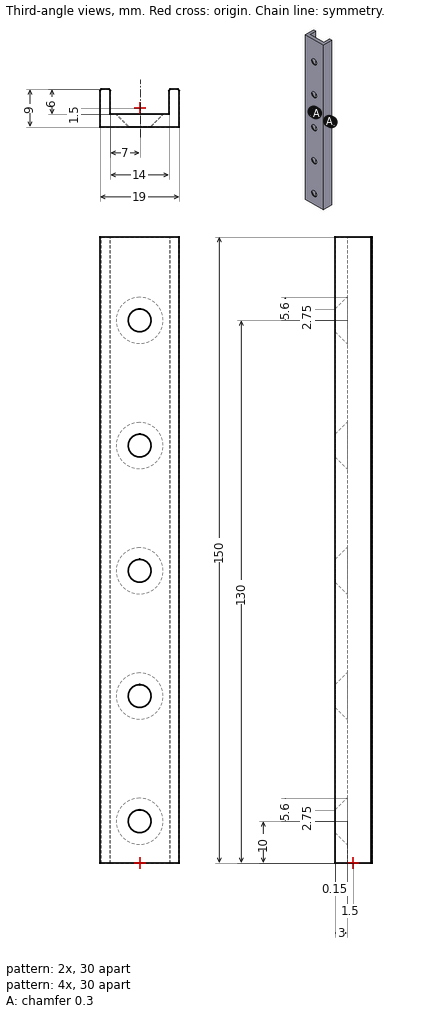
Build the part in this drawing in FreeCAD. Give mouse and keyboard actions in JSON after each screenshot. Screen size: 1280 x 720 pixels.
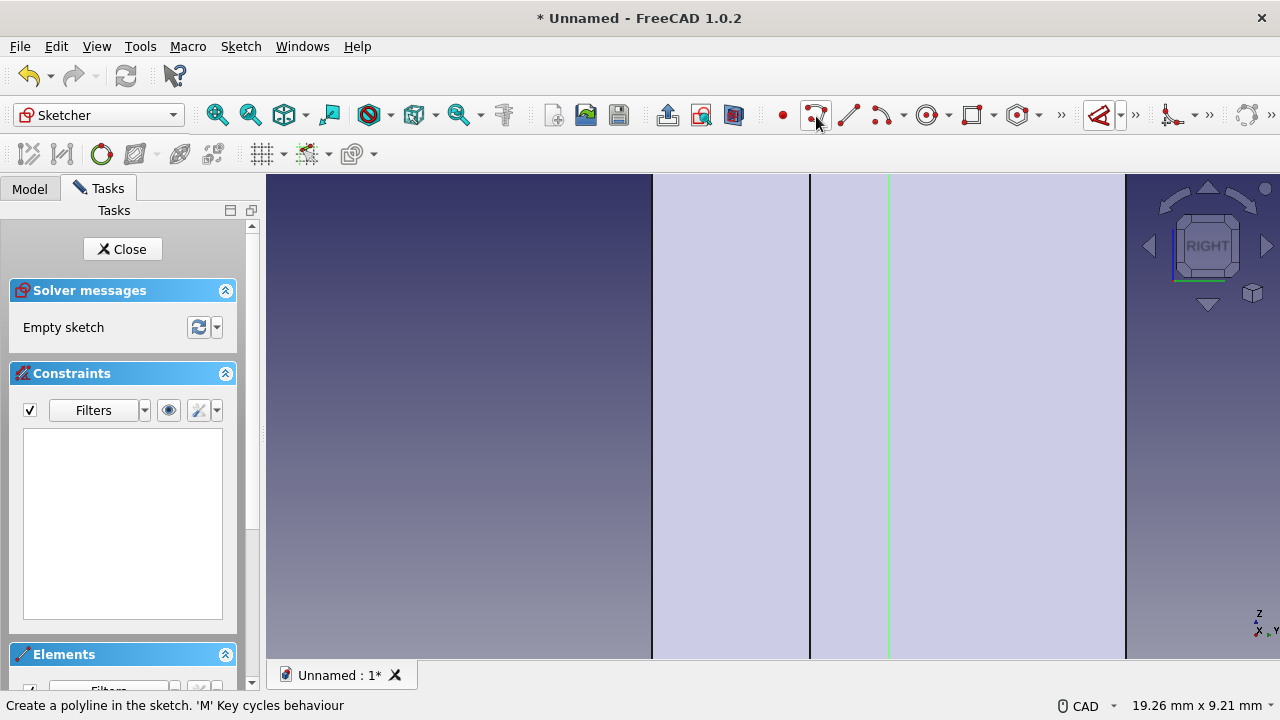
{"action": "left_click", "coordinate": [810, 569]}
{"action": "left_click", "coordinate": [810, 274]}
{"action": "left_click", "coordinate": [660, 424]}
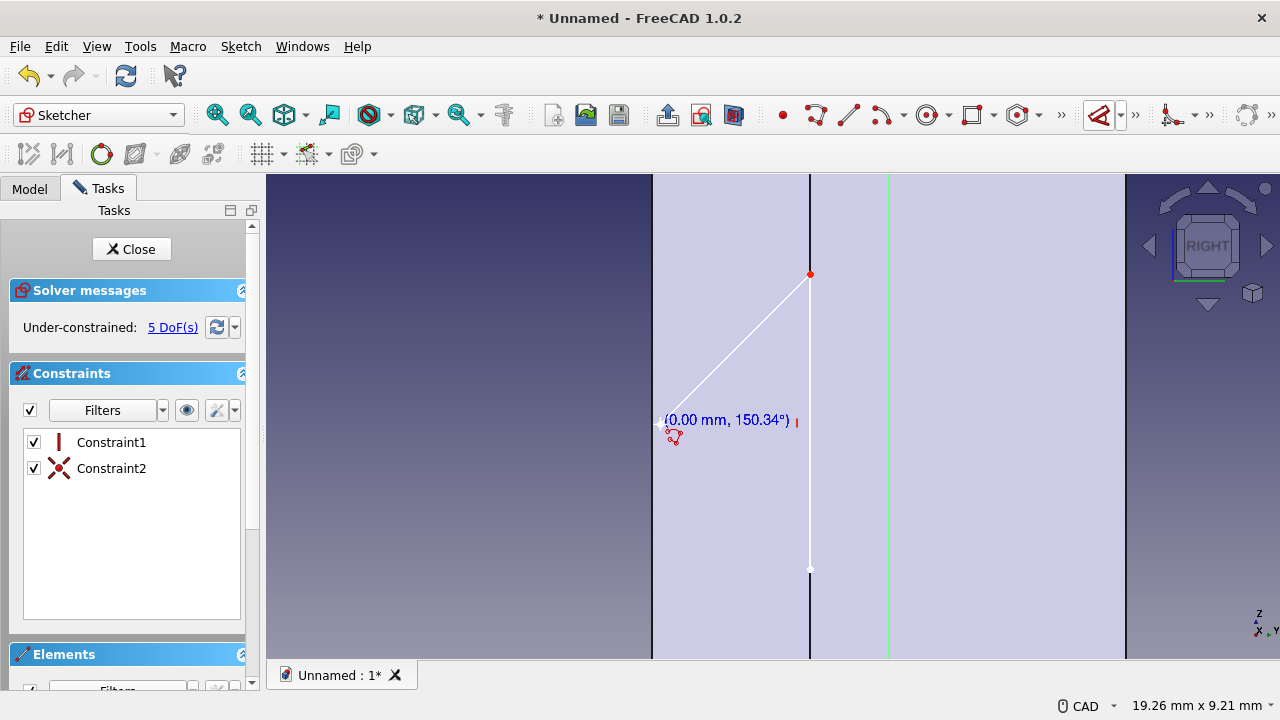
{"action": "scroll", "coordinate": [652, 424], "scroll_direction": "up", "scroll_amount": 4}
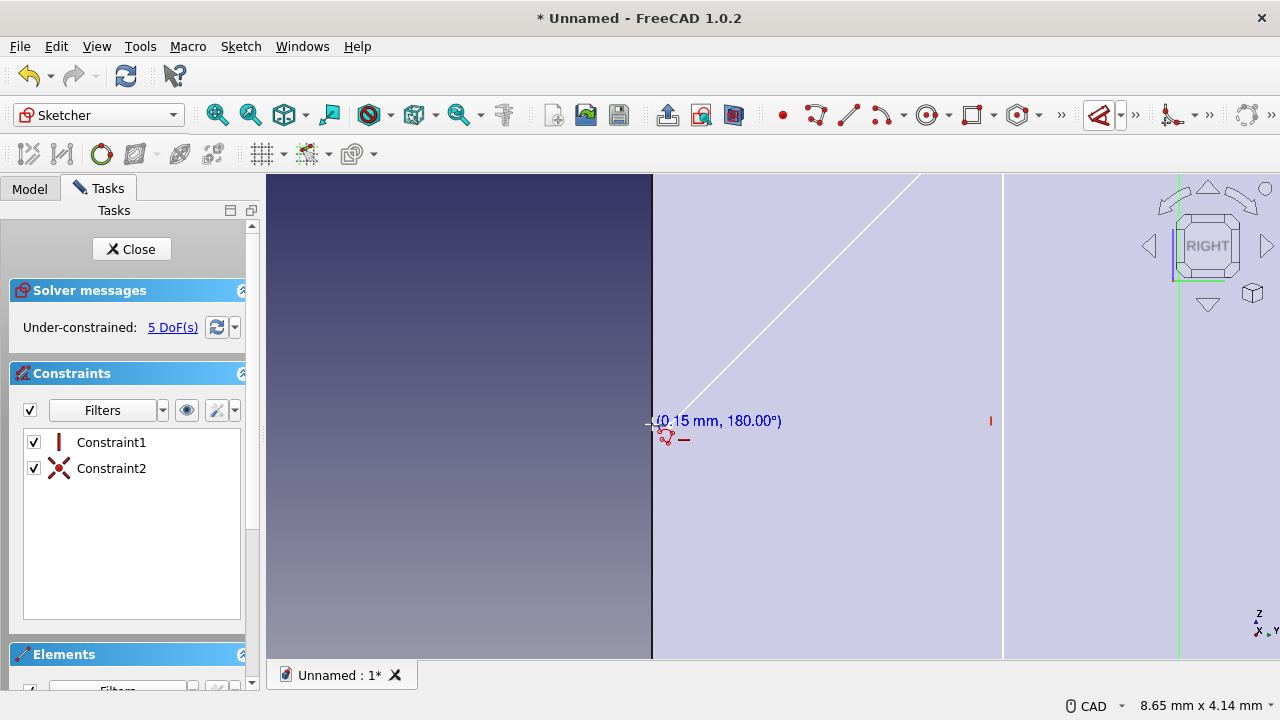
{"action": "left_click", "coordinate": [652, 423]}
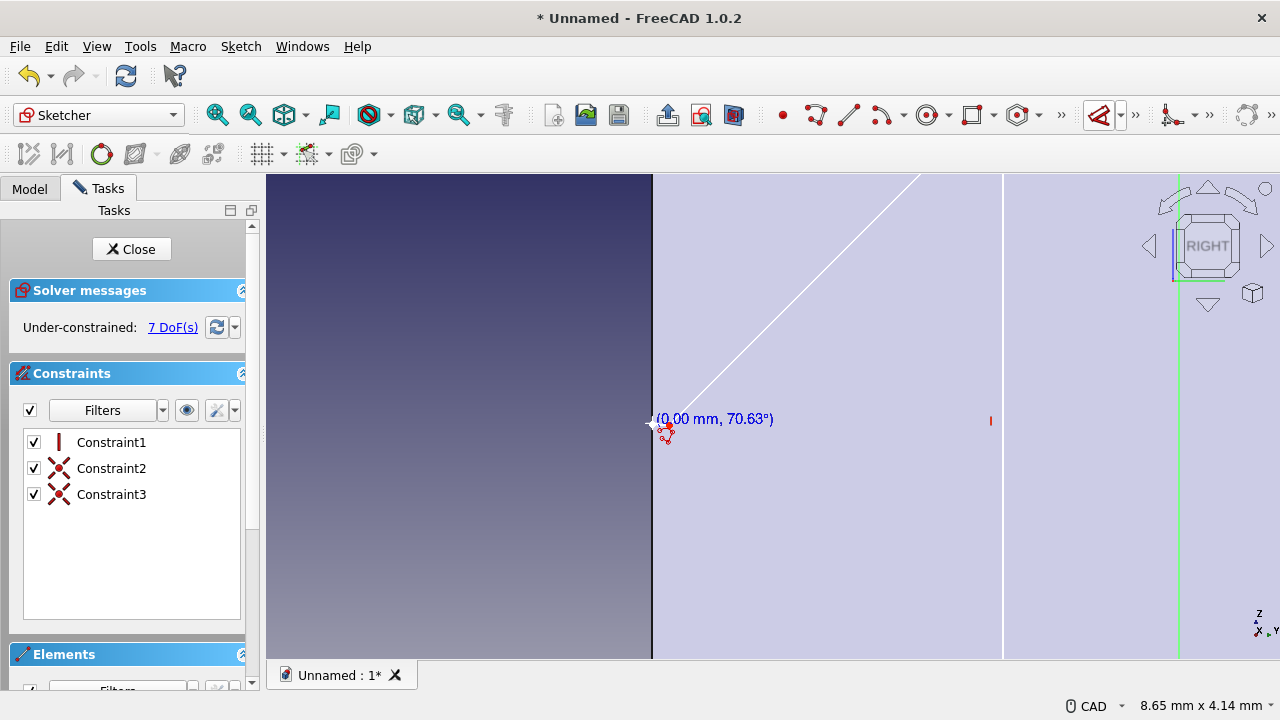
{"action": "scroll", "coordinate": [662, 415], "scroll_direction": "down", "scroll_amount": 4}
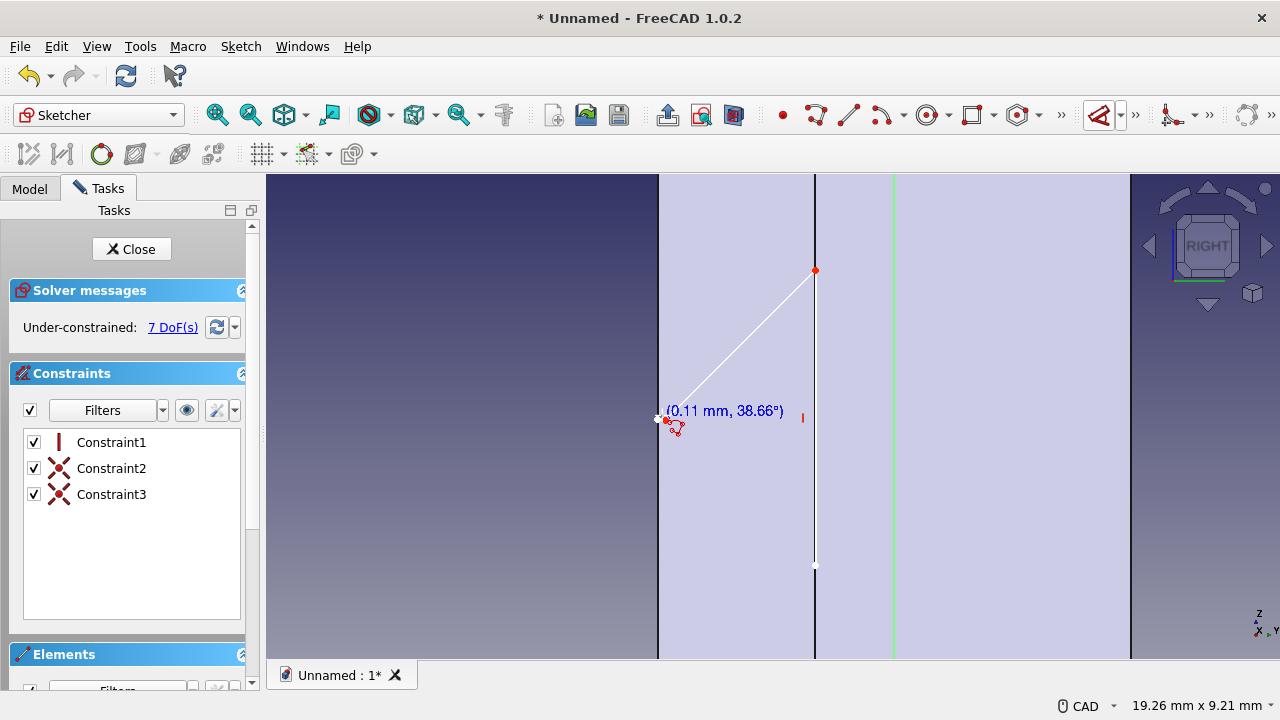
{"action": "left_click", "coordinate": [658, 564]}
{"action": "left_click", "coordinate": [816, 565]}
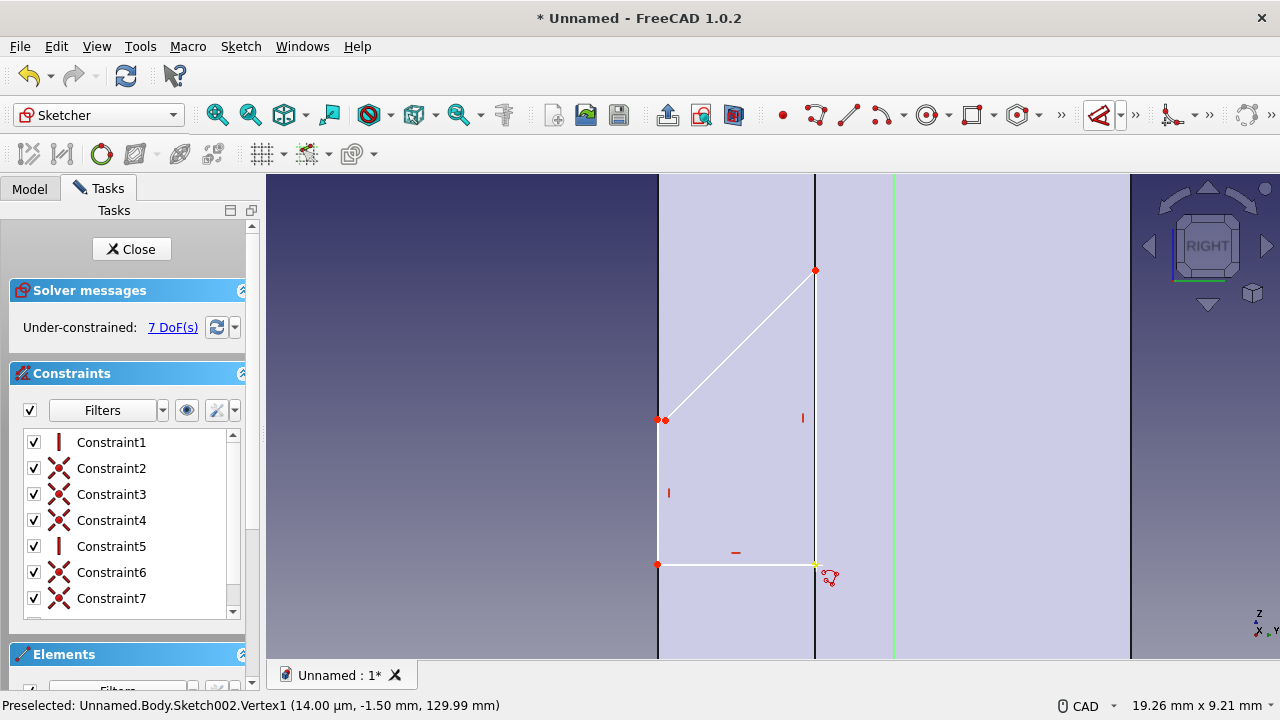
{"action": "left_click", "coordinate": [849, 116]}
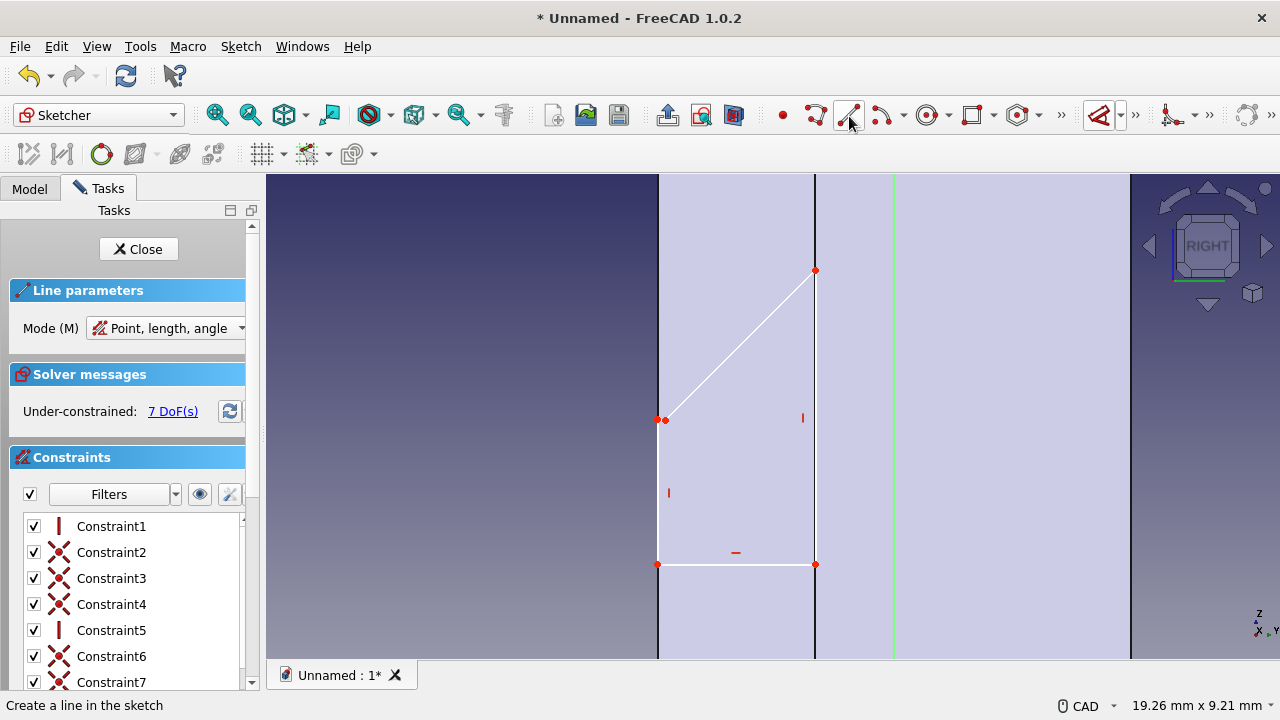
{"action": "left_click", "coordinate": [642, 564]}
{"action": "left_click", "coordinate": [594, 564]}
{"action": "key", "text": "Escape"}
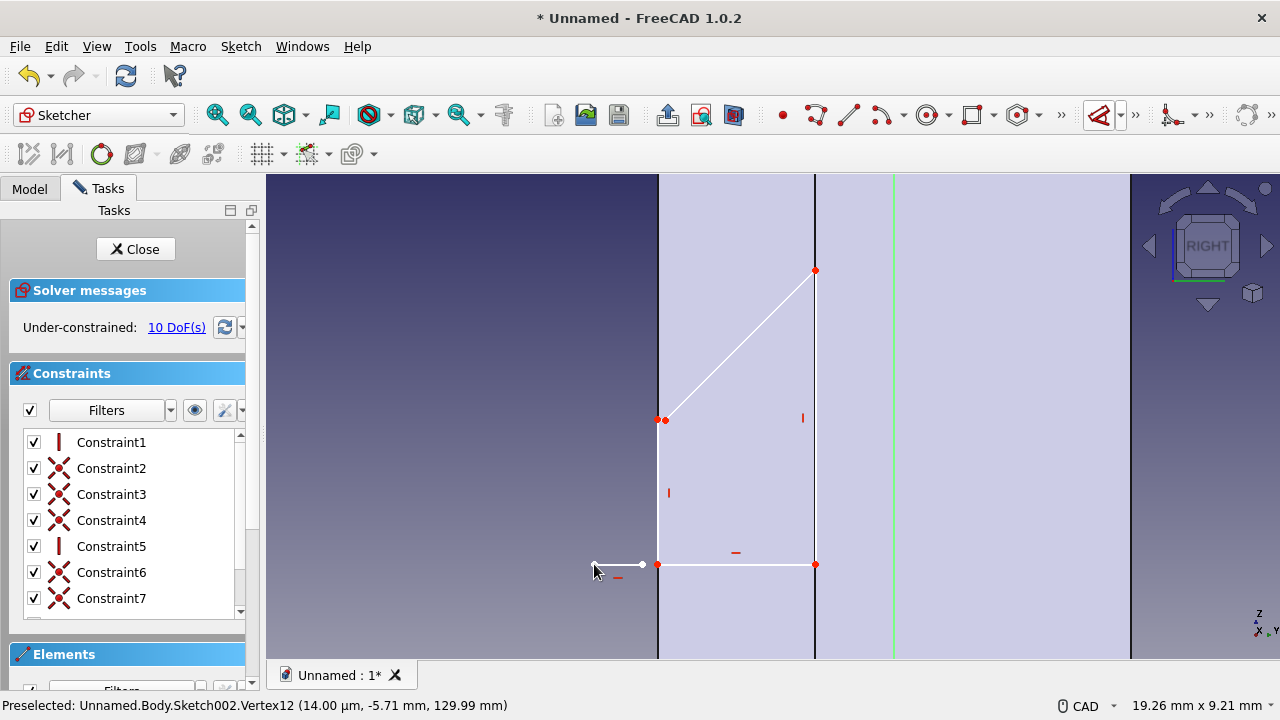
{"action": "left_click", "coordinate": [628, 565]}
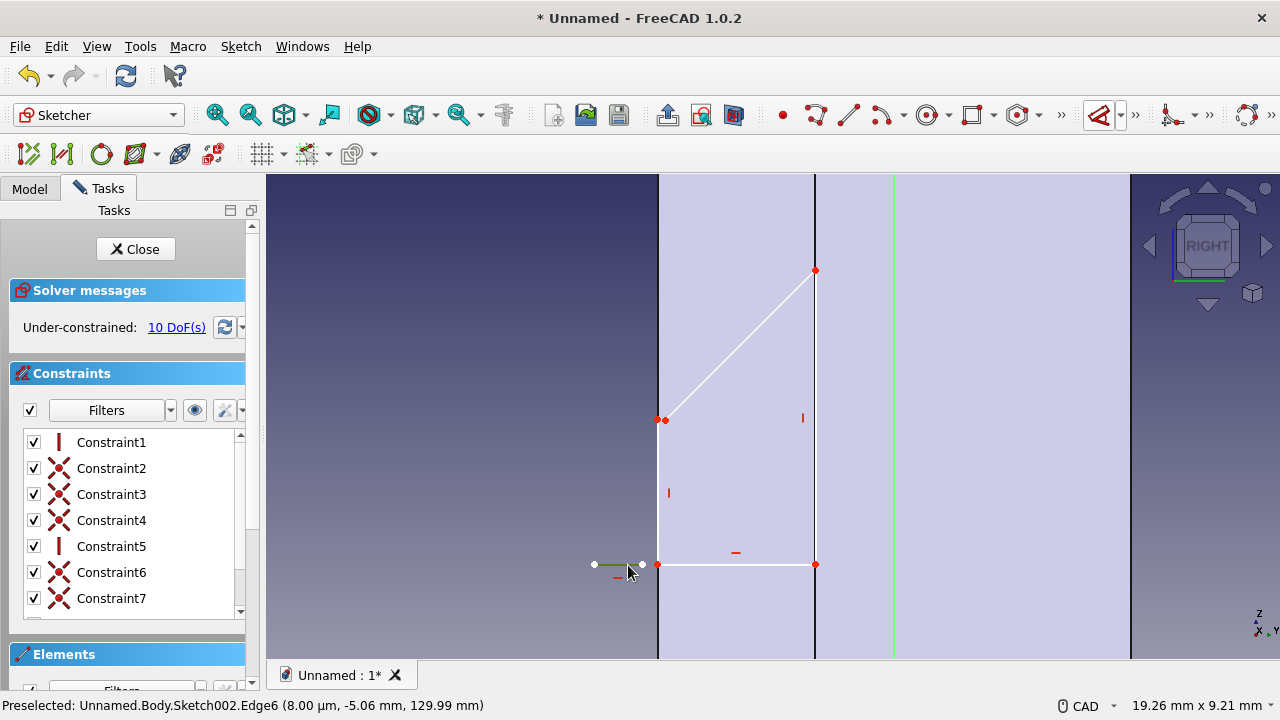
{"action": "key", "text": "g n"}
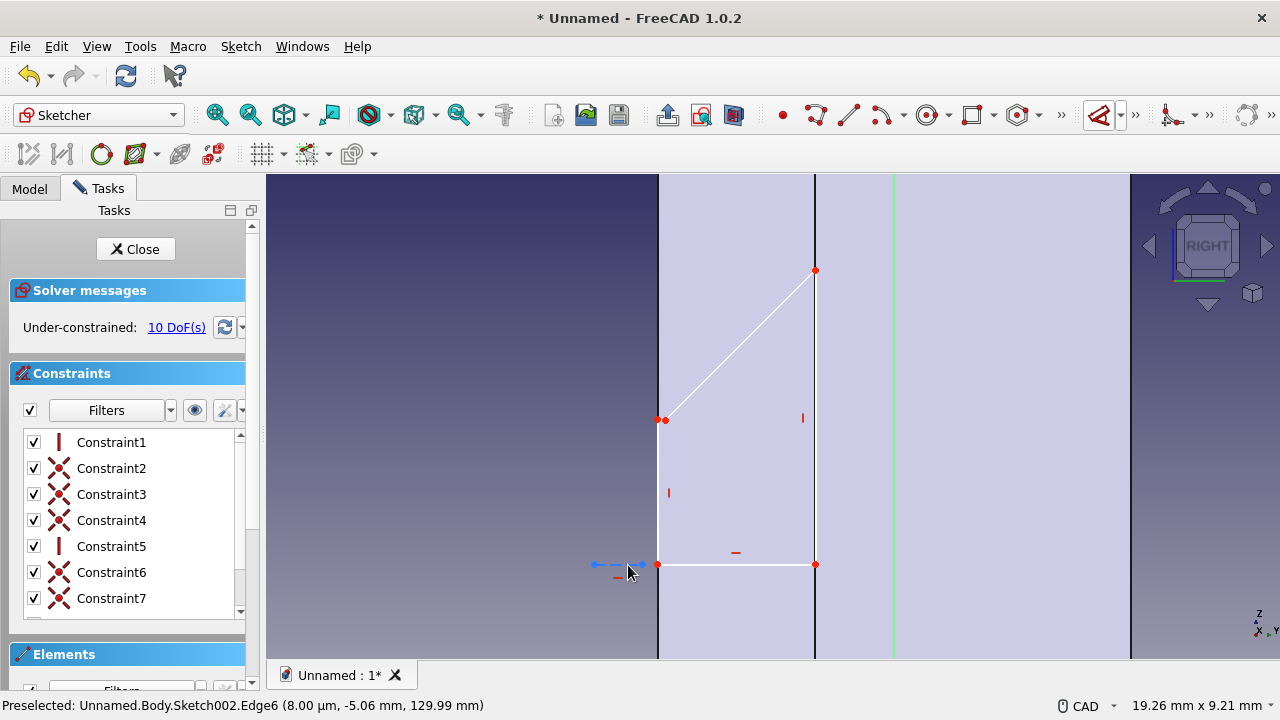
{"action": "scroll", "coordinate": [662, 420], "scroll_direction": "up", "scroll_amount": 7}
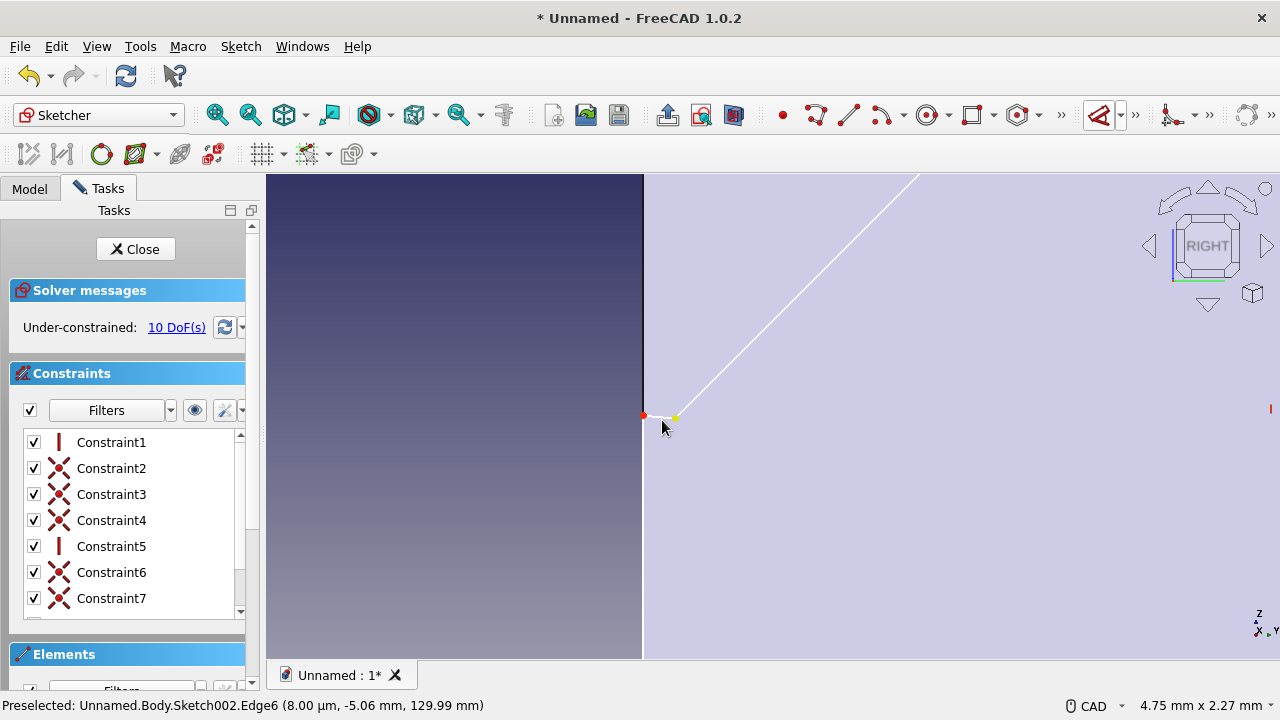
{"action": "left_click", "coordinate": [659, 417]}